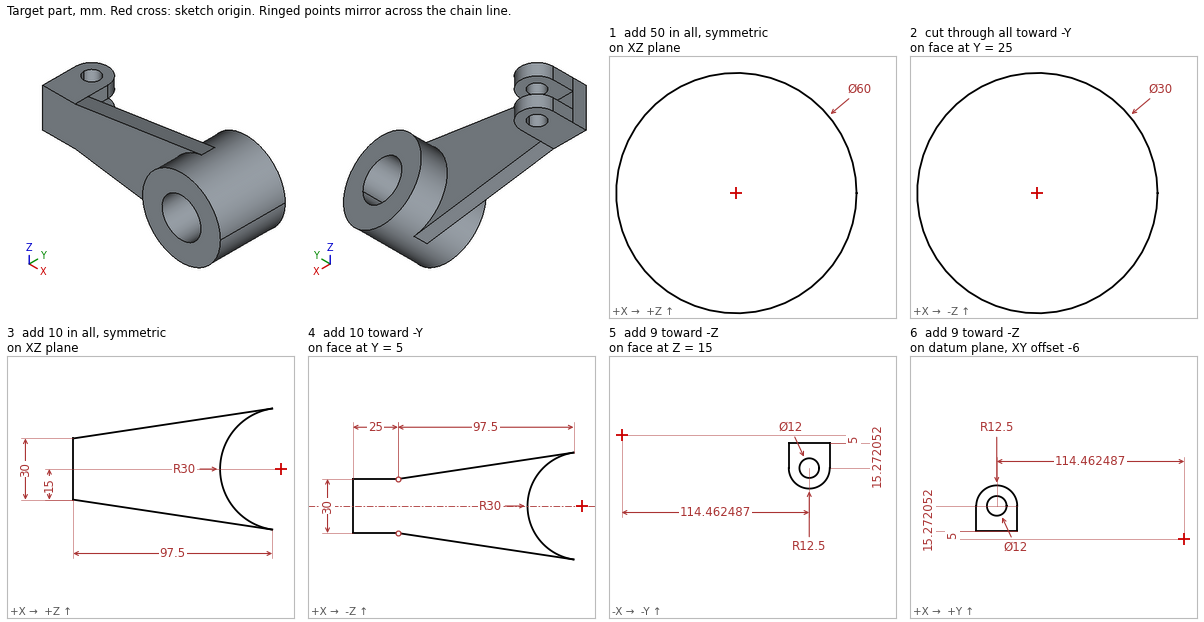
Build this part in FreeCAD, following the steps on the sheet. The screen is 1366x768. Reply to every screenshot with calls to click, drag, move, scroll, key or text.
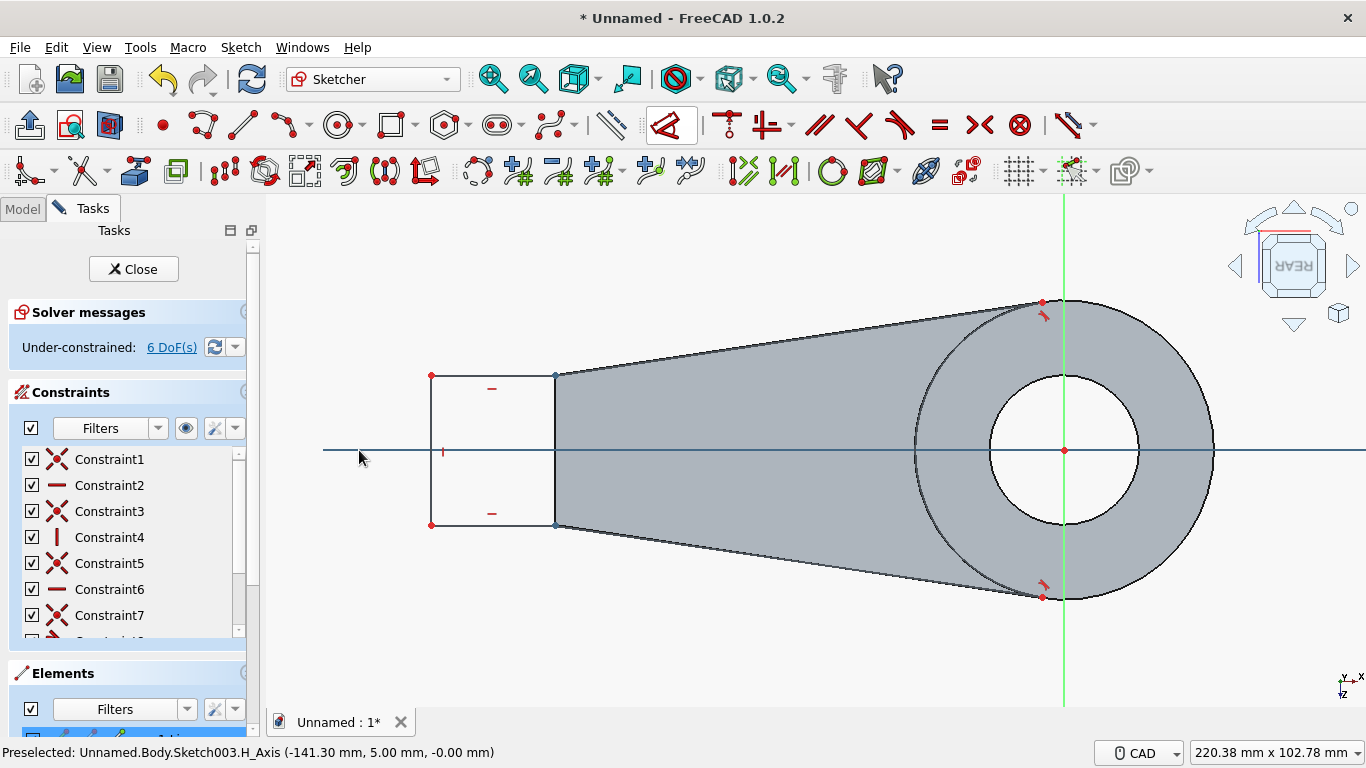
click(980, 126)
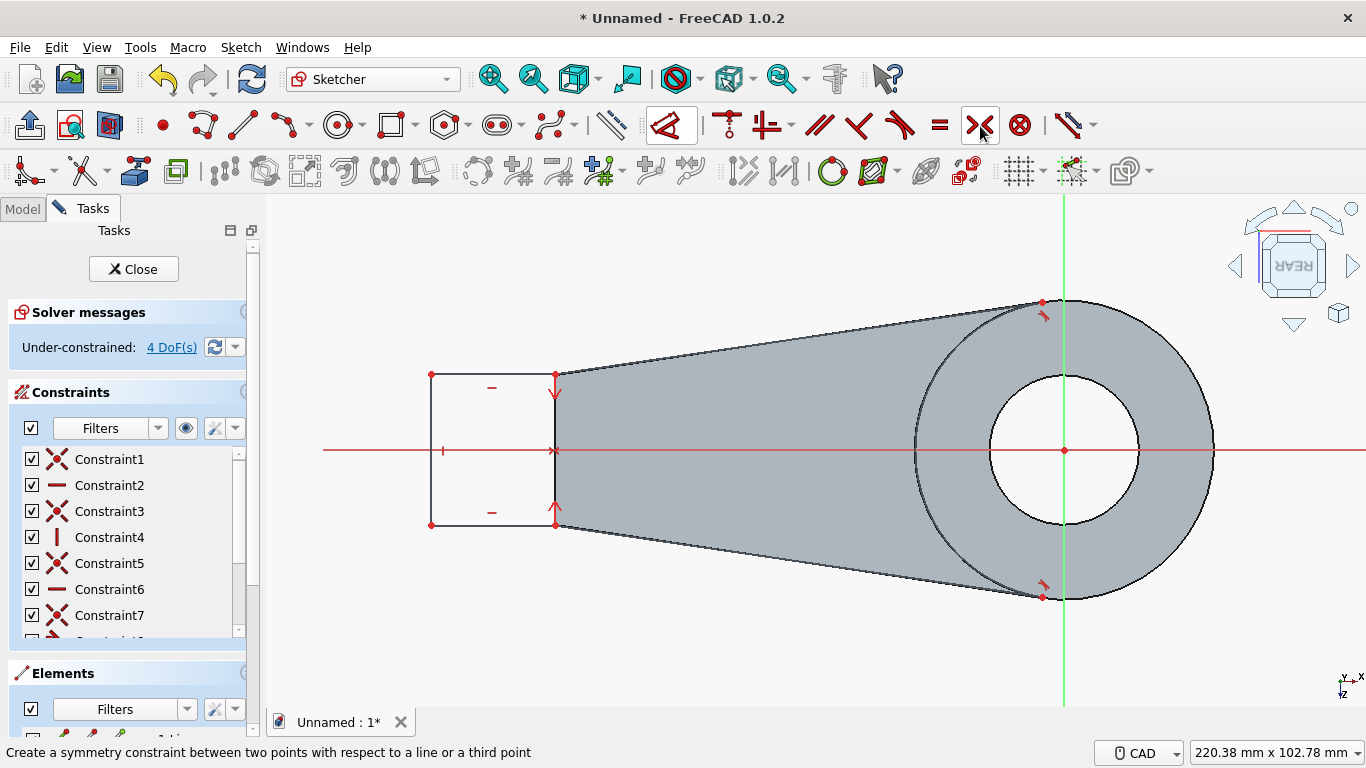
click(939, 370)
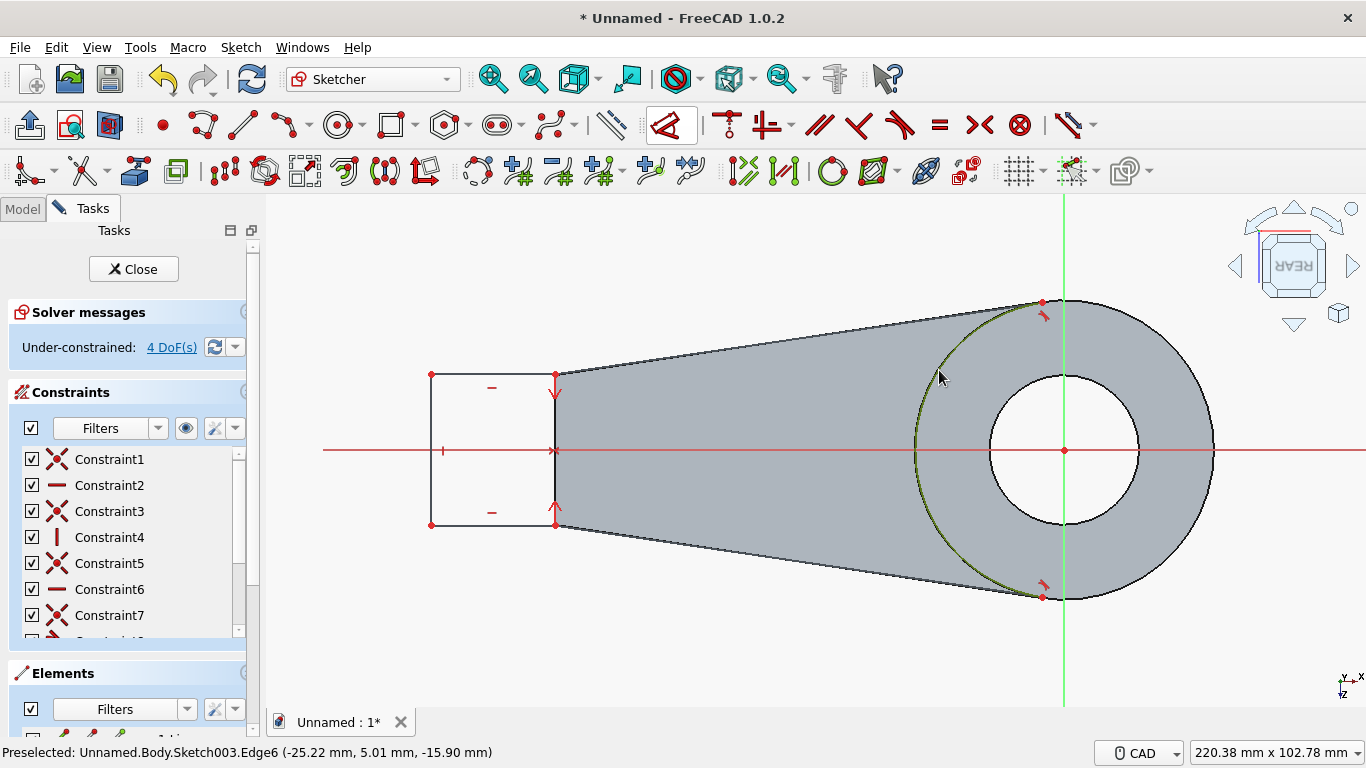
click(692, 126)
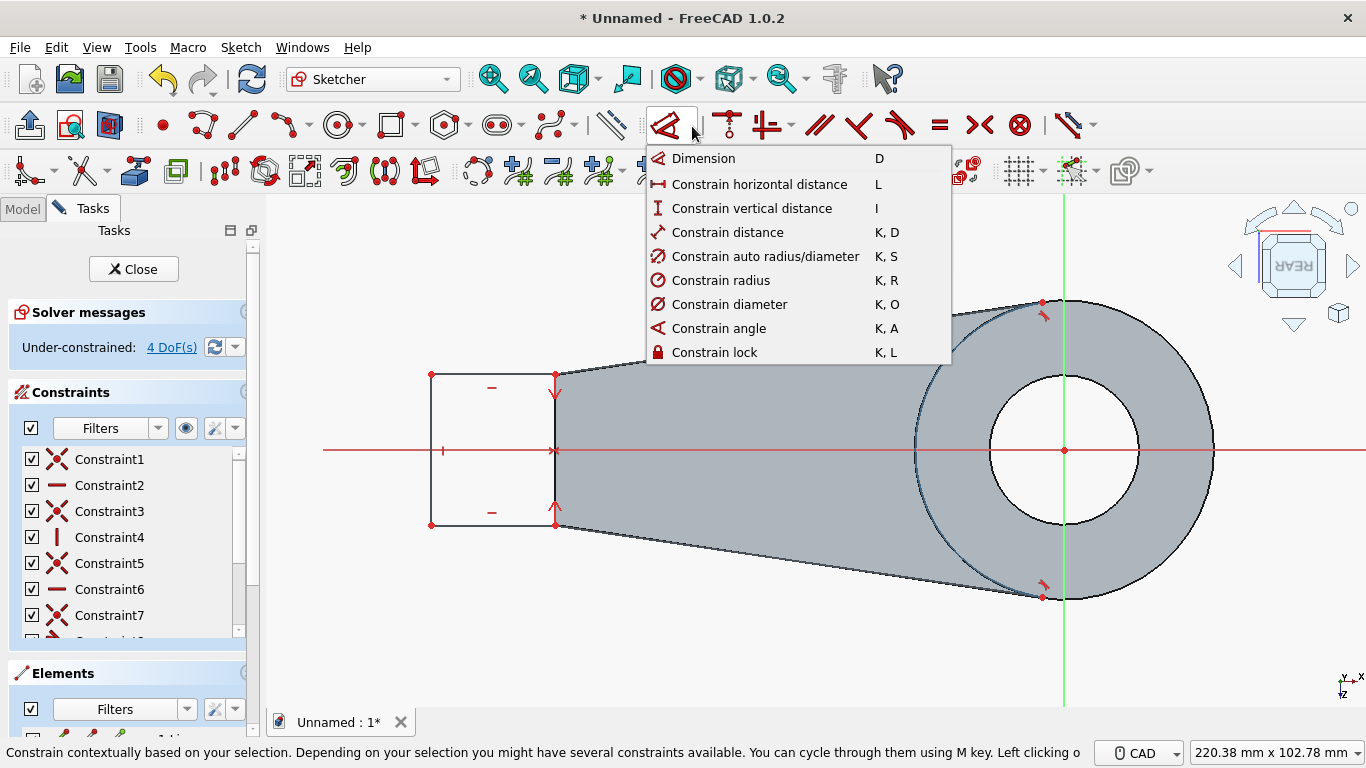
click(799, 280)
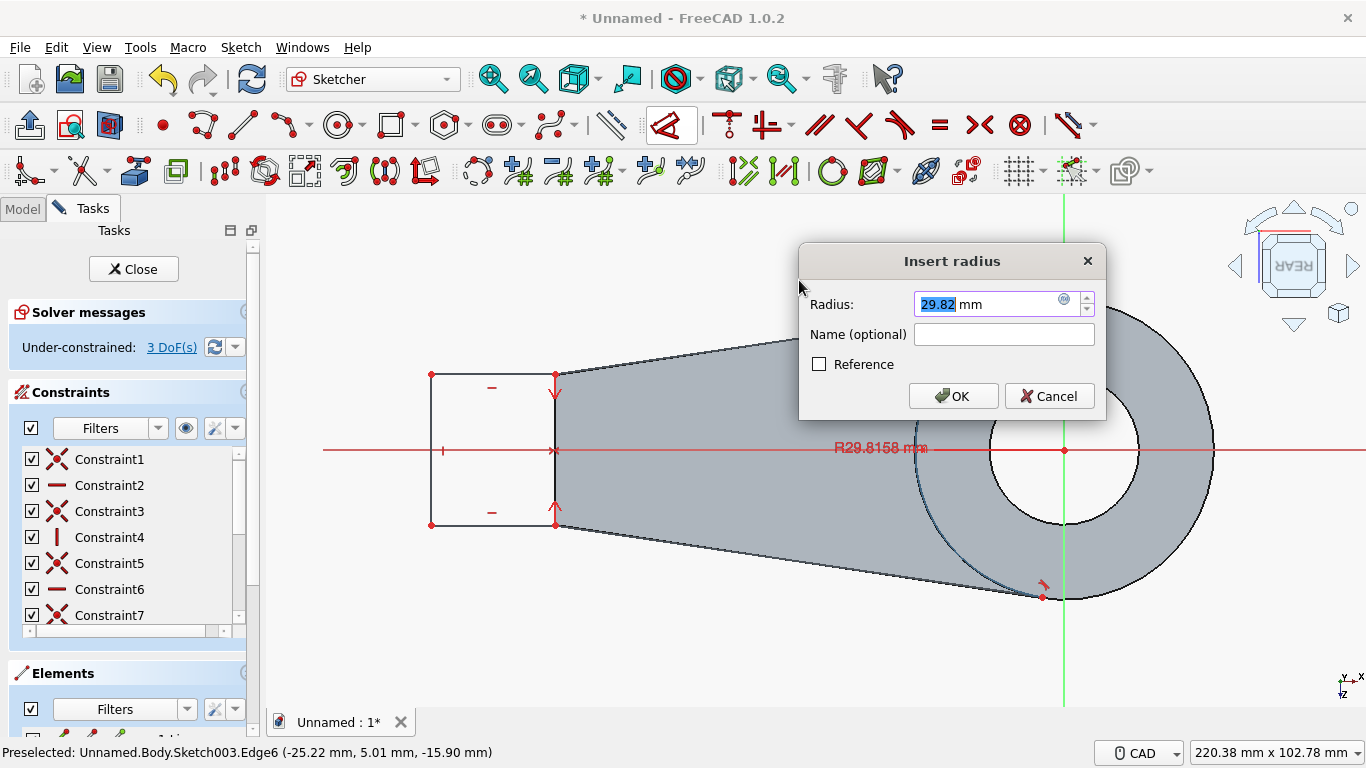
text(30)
key(Return)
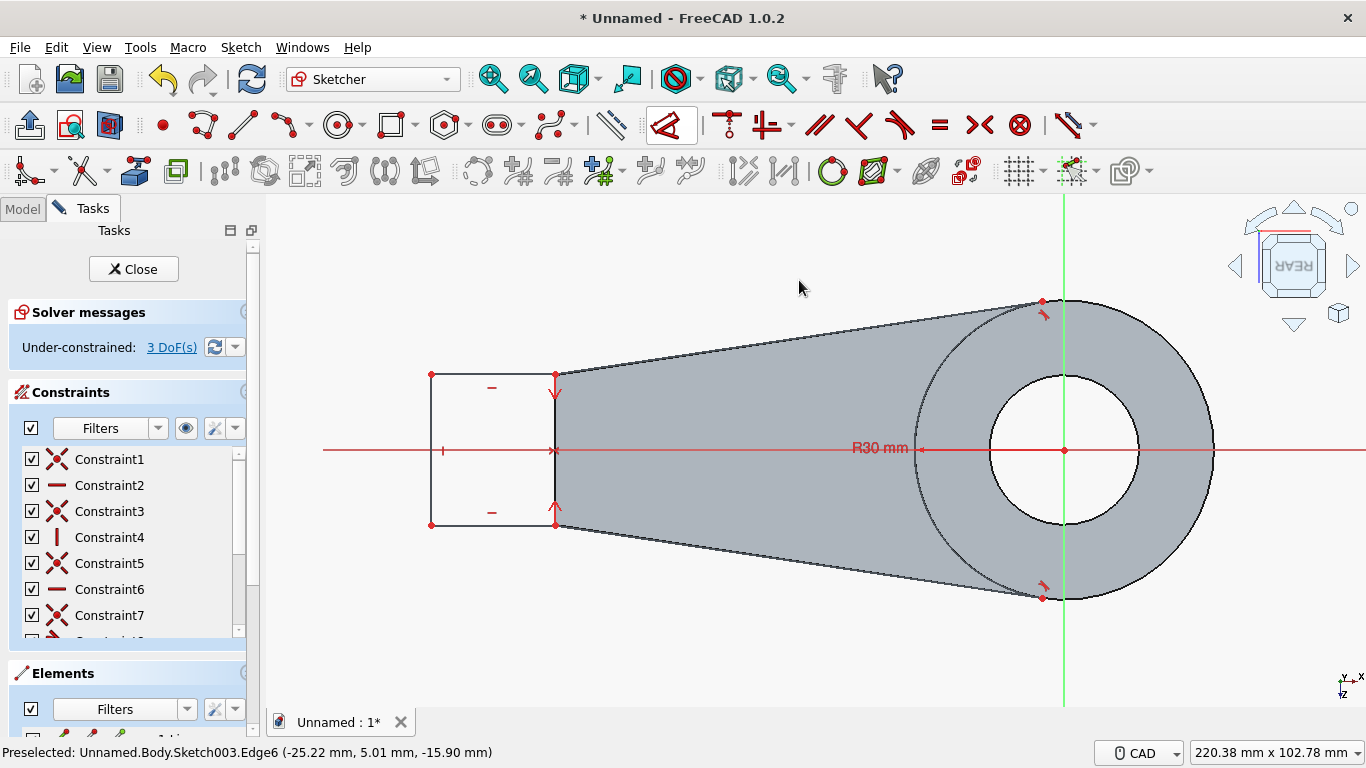
click(518, 374)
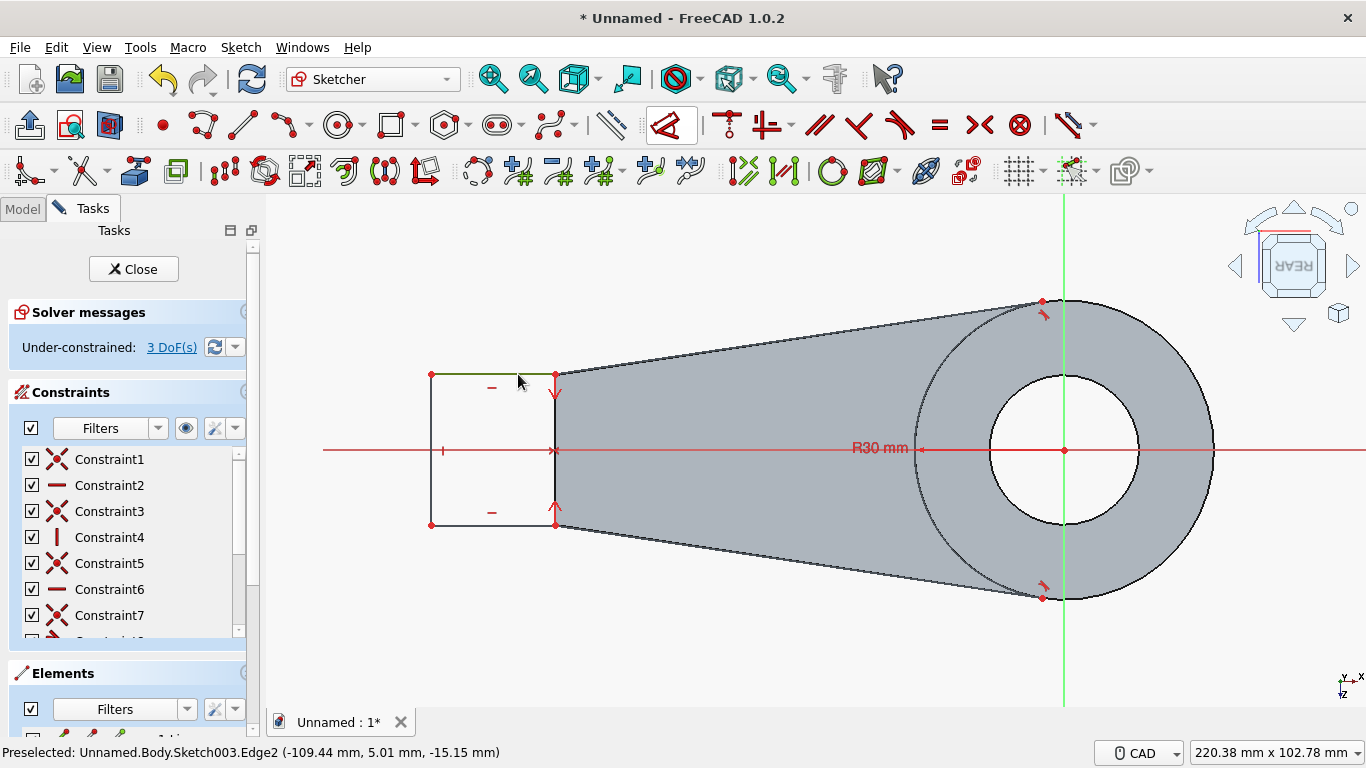
key(l)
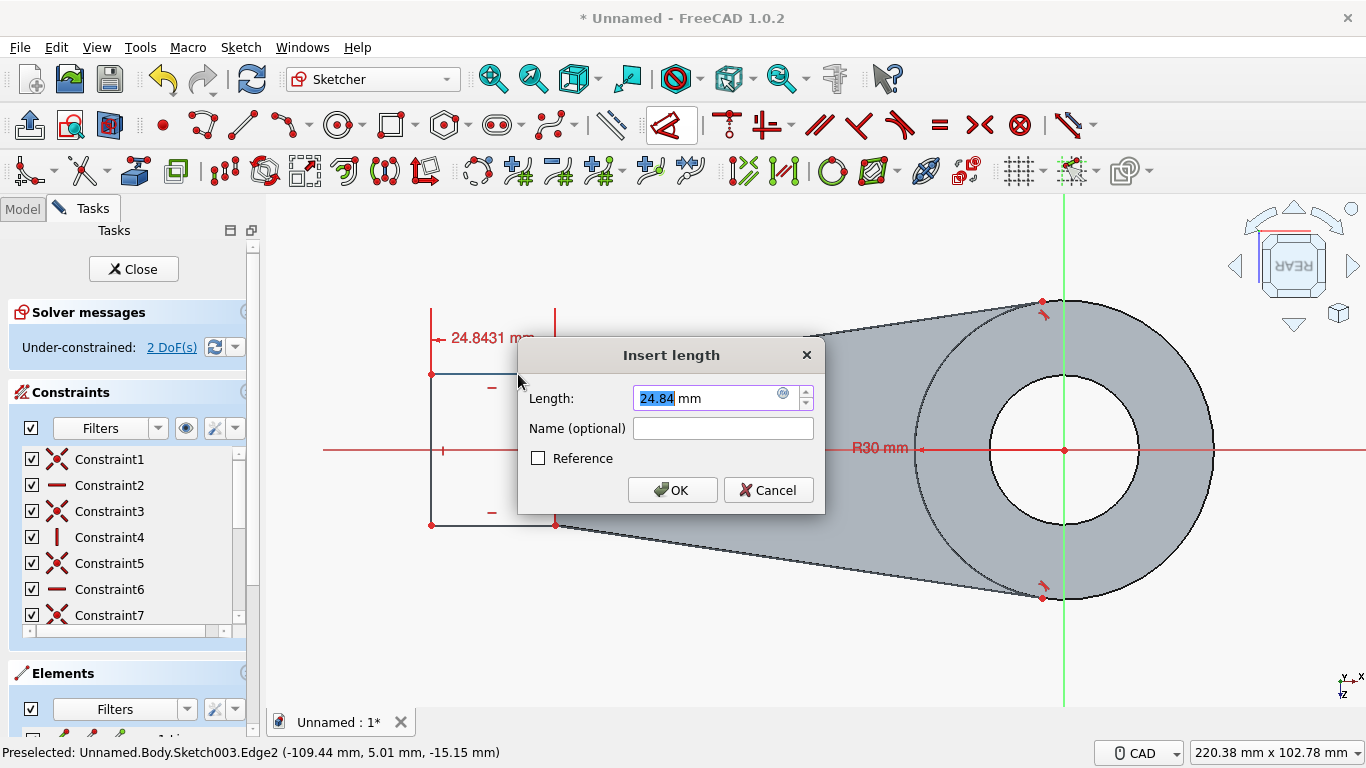
text(25)
key(Return)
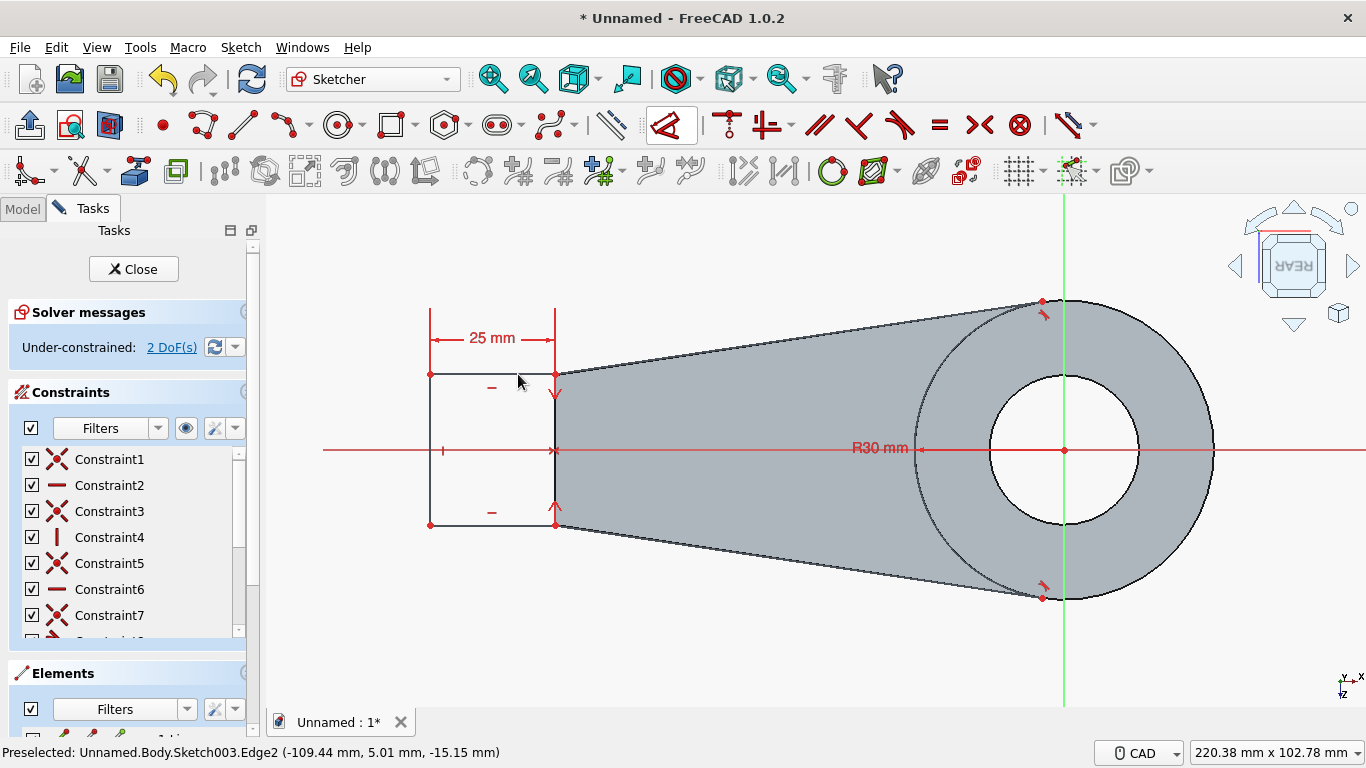
click(430, 420)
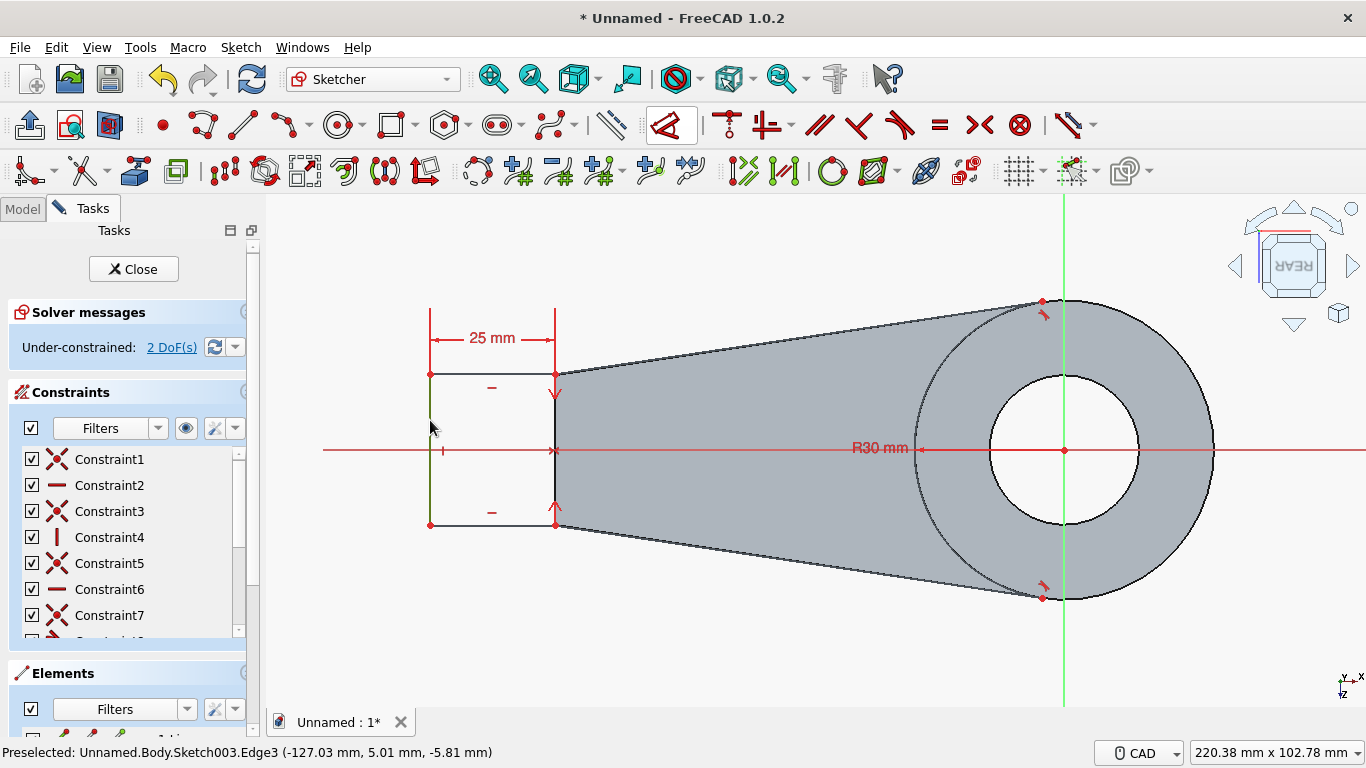
key(i)